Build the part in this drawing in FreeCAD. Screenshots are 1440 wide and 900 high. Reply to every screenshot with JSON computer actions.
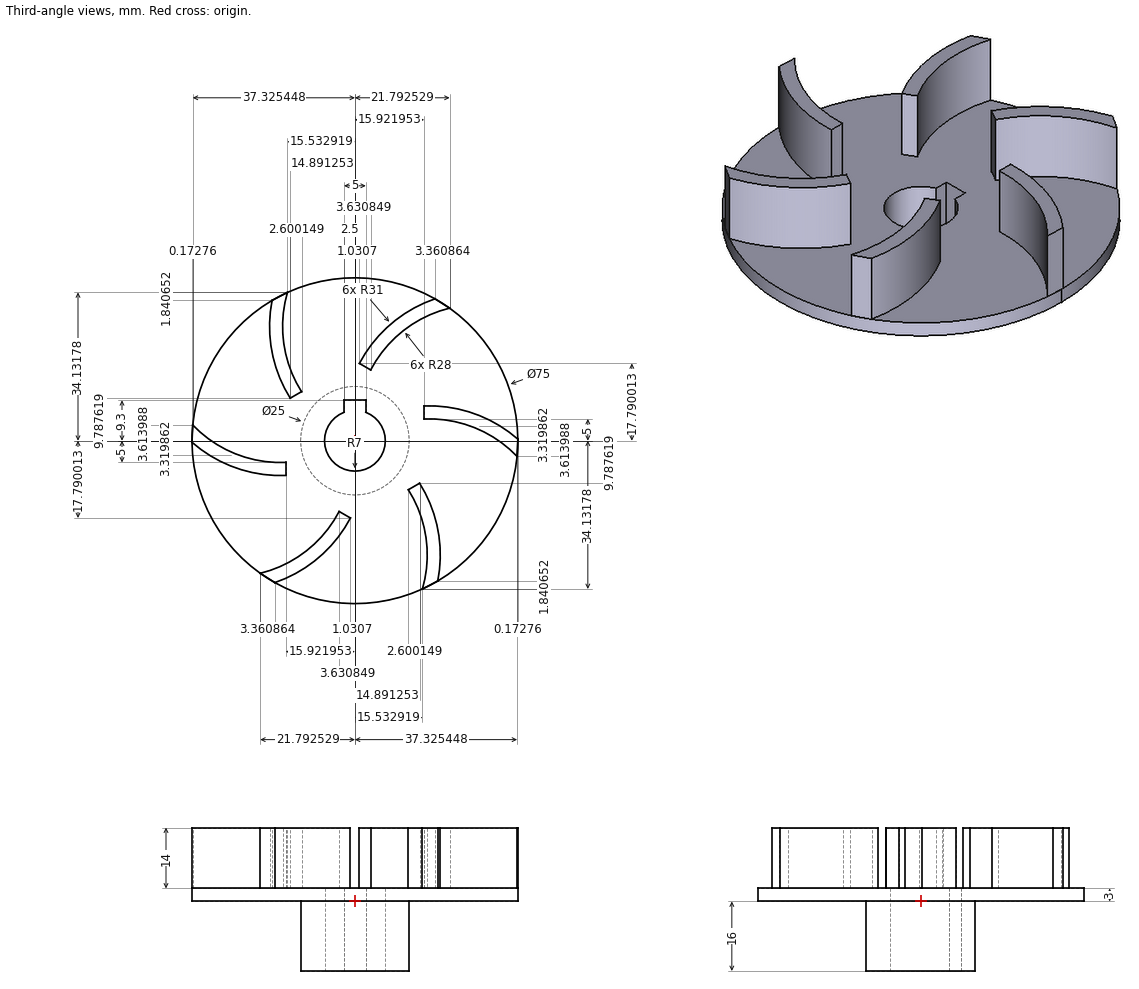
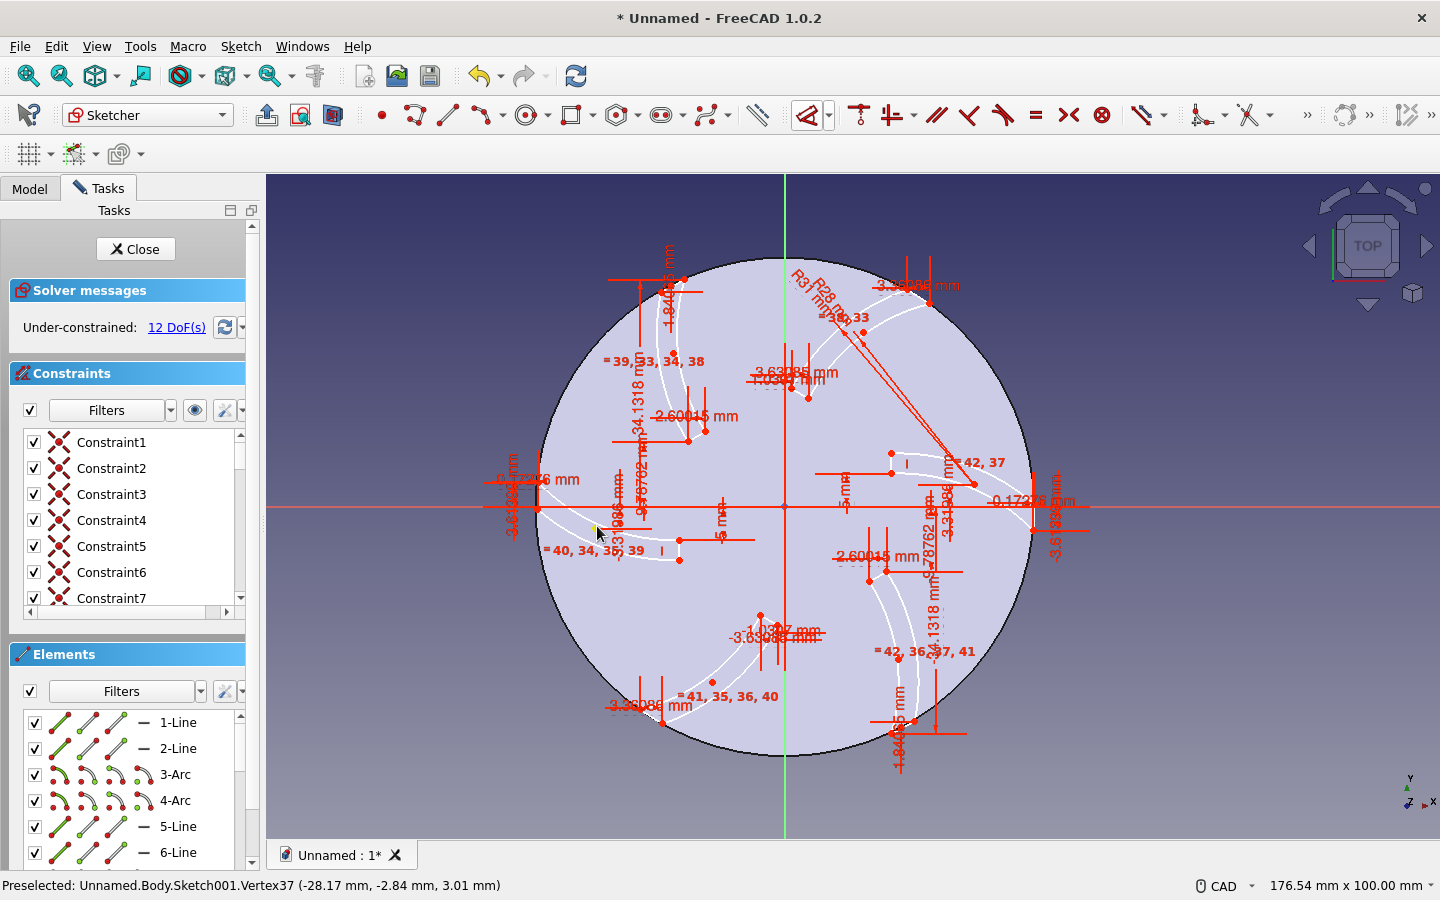
{"action": "left_click", "coordinate": [930, 304]}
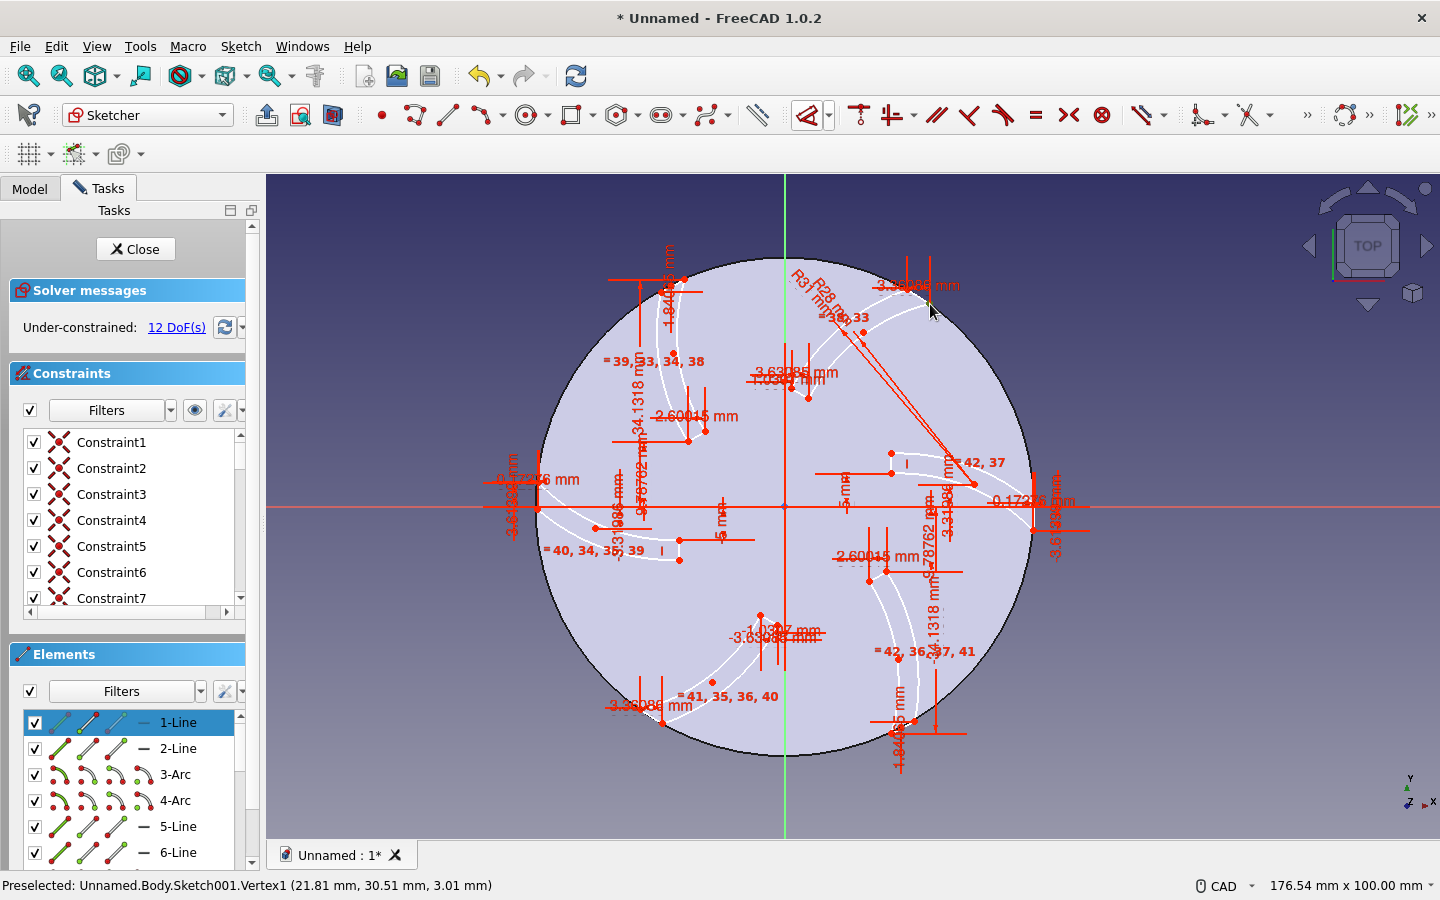
{"action": "left_click", "coordinate": [828, 116]}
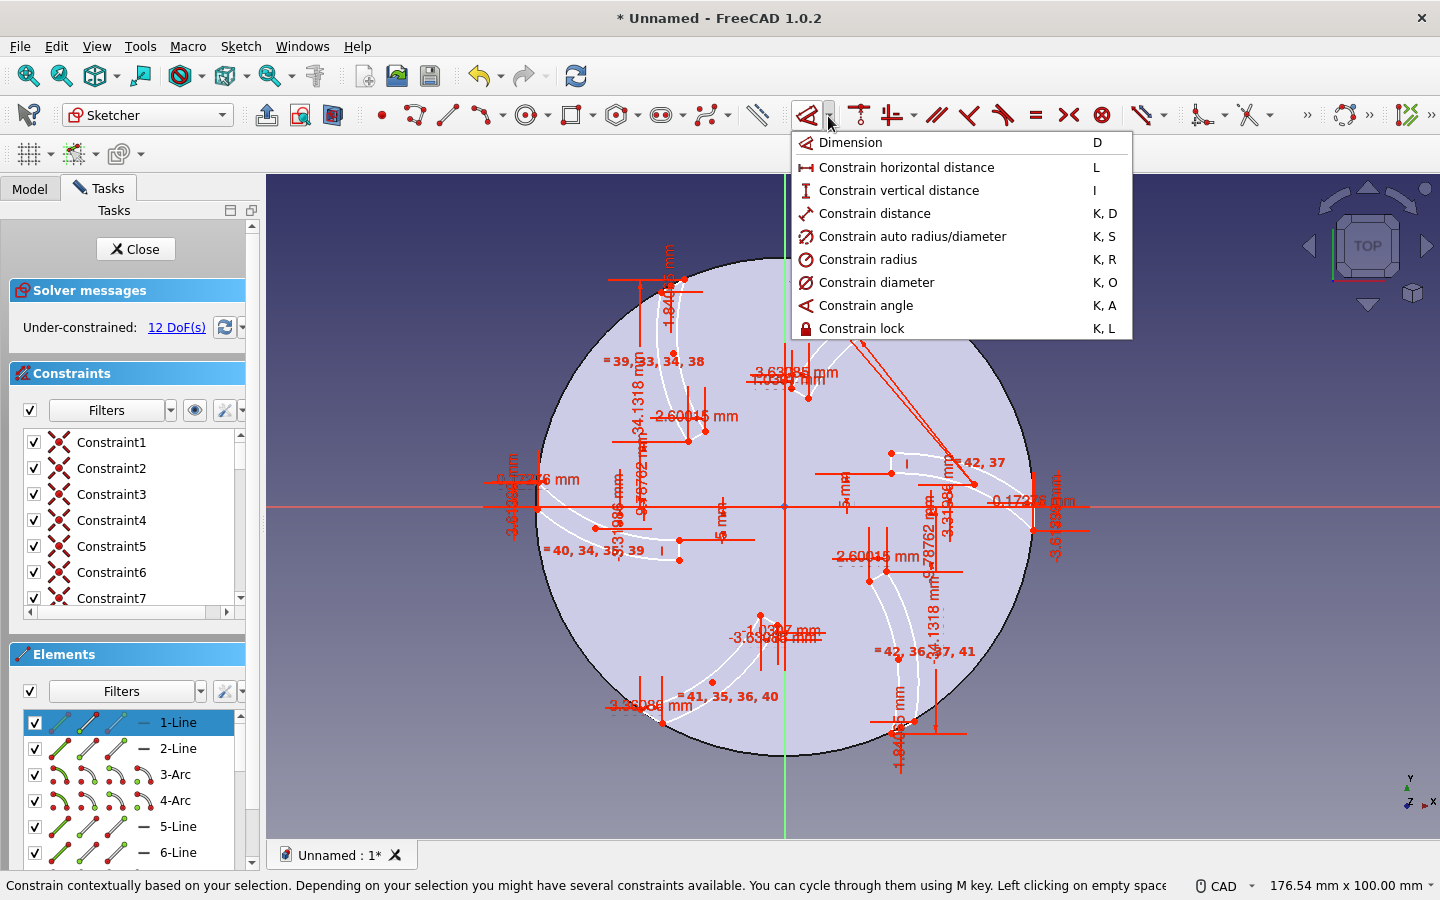
{"action": "left_click", "coordinate": [962, 168]}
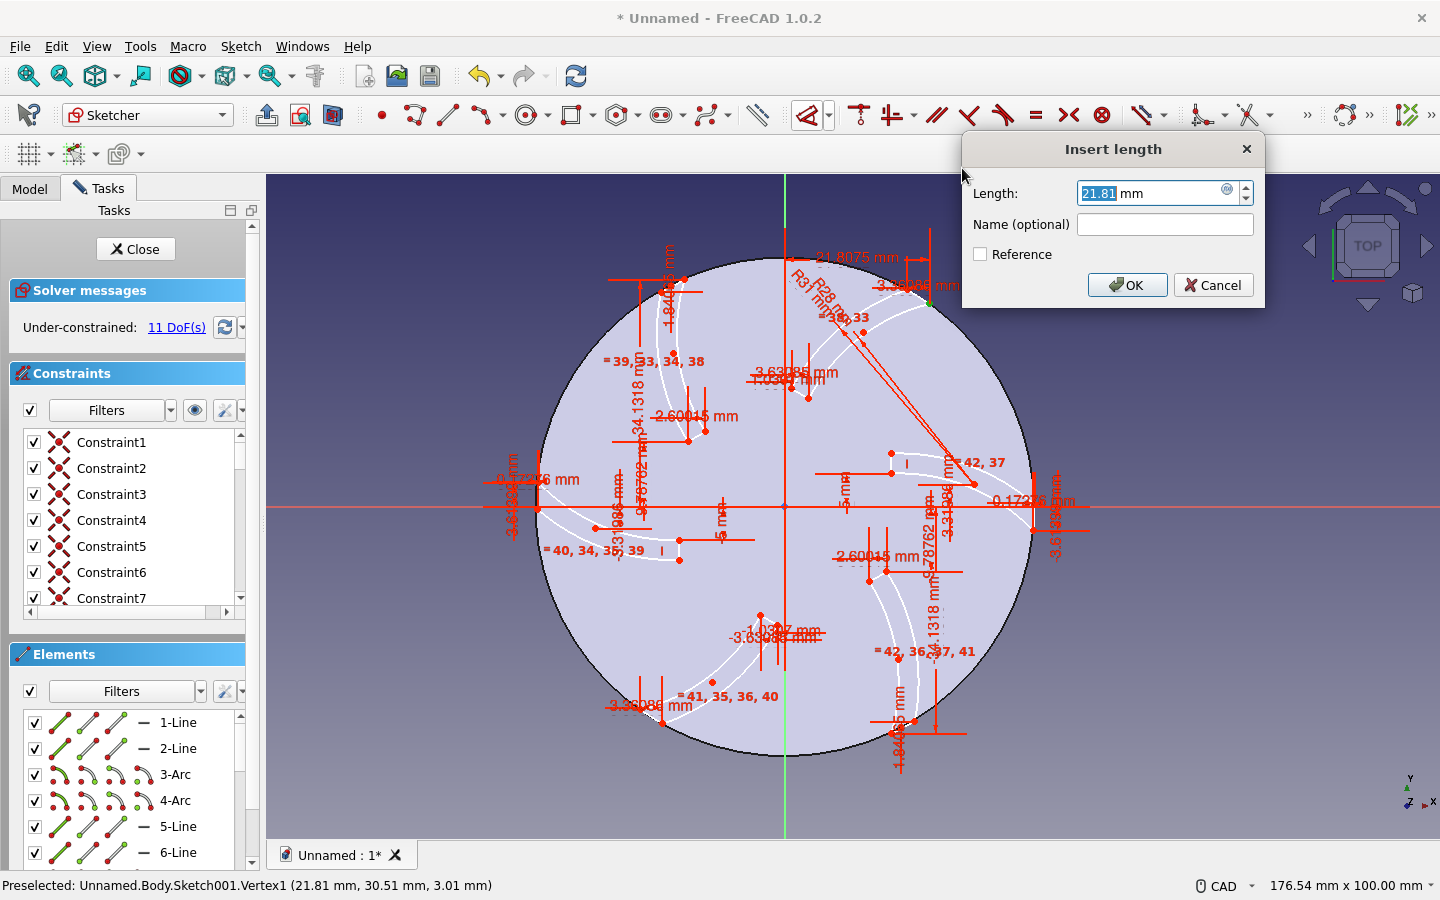
{"action": "type", "text": "21.792529"}
{"action": "key", "text": "Return"}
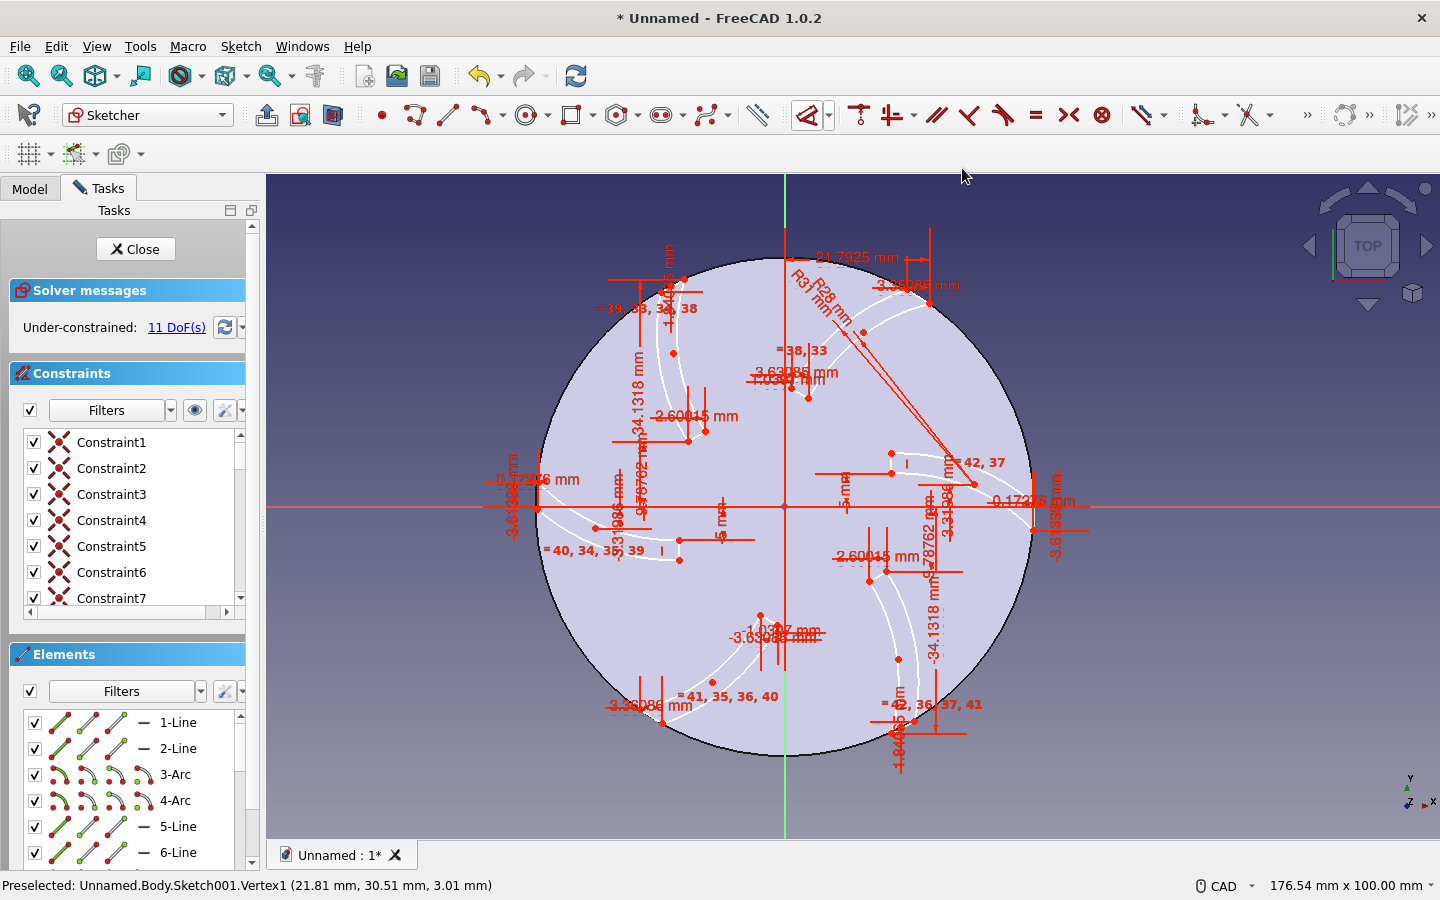
{"action": "left_click", "coordinate": [792, 389]}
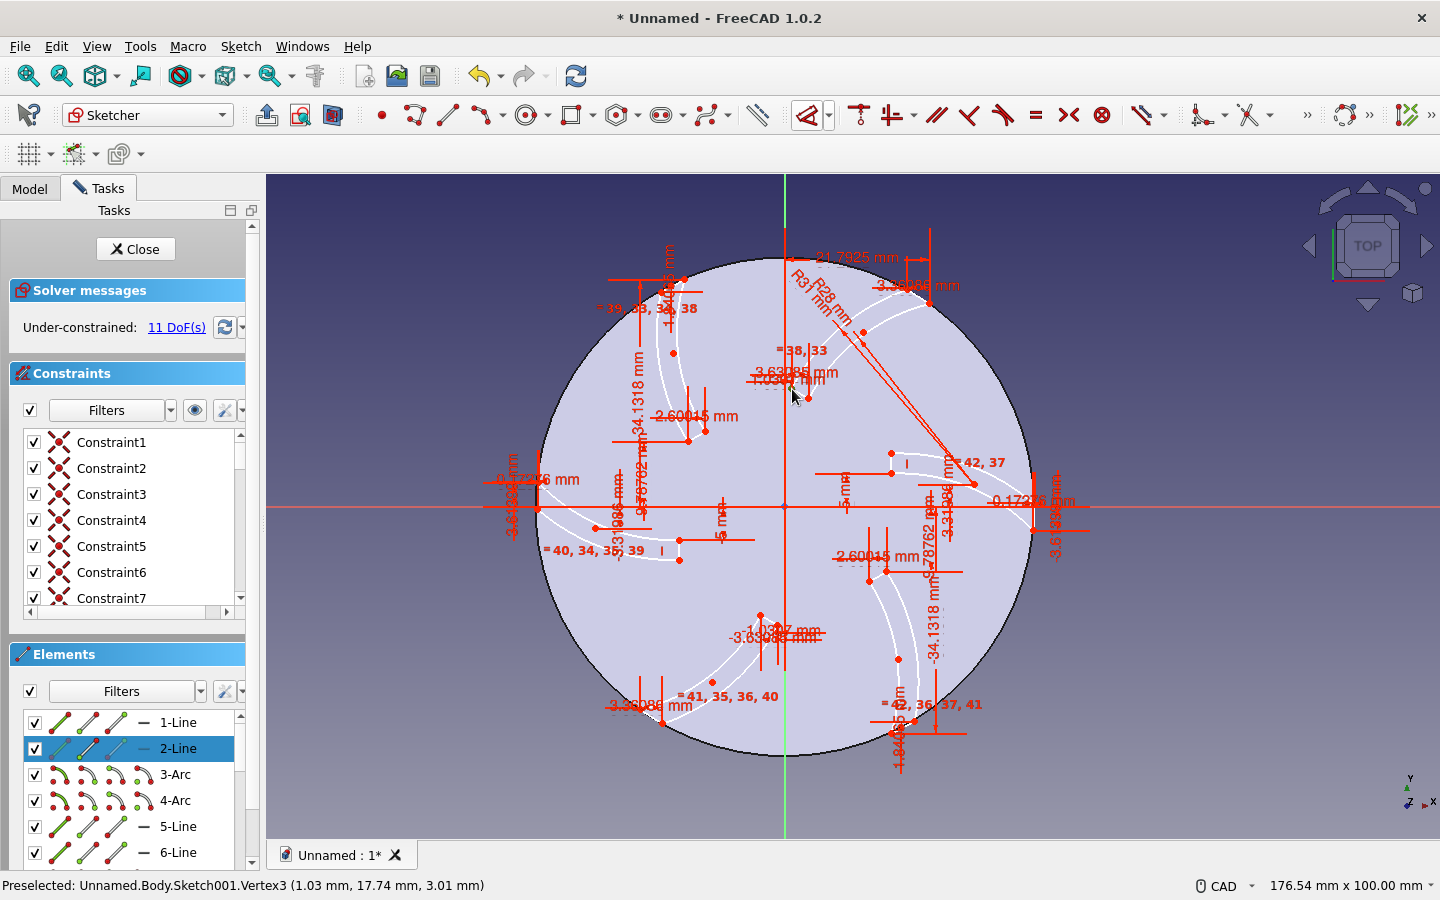
{"action": "key", "text": "i"}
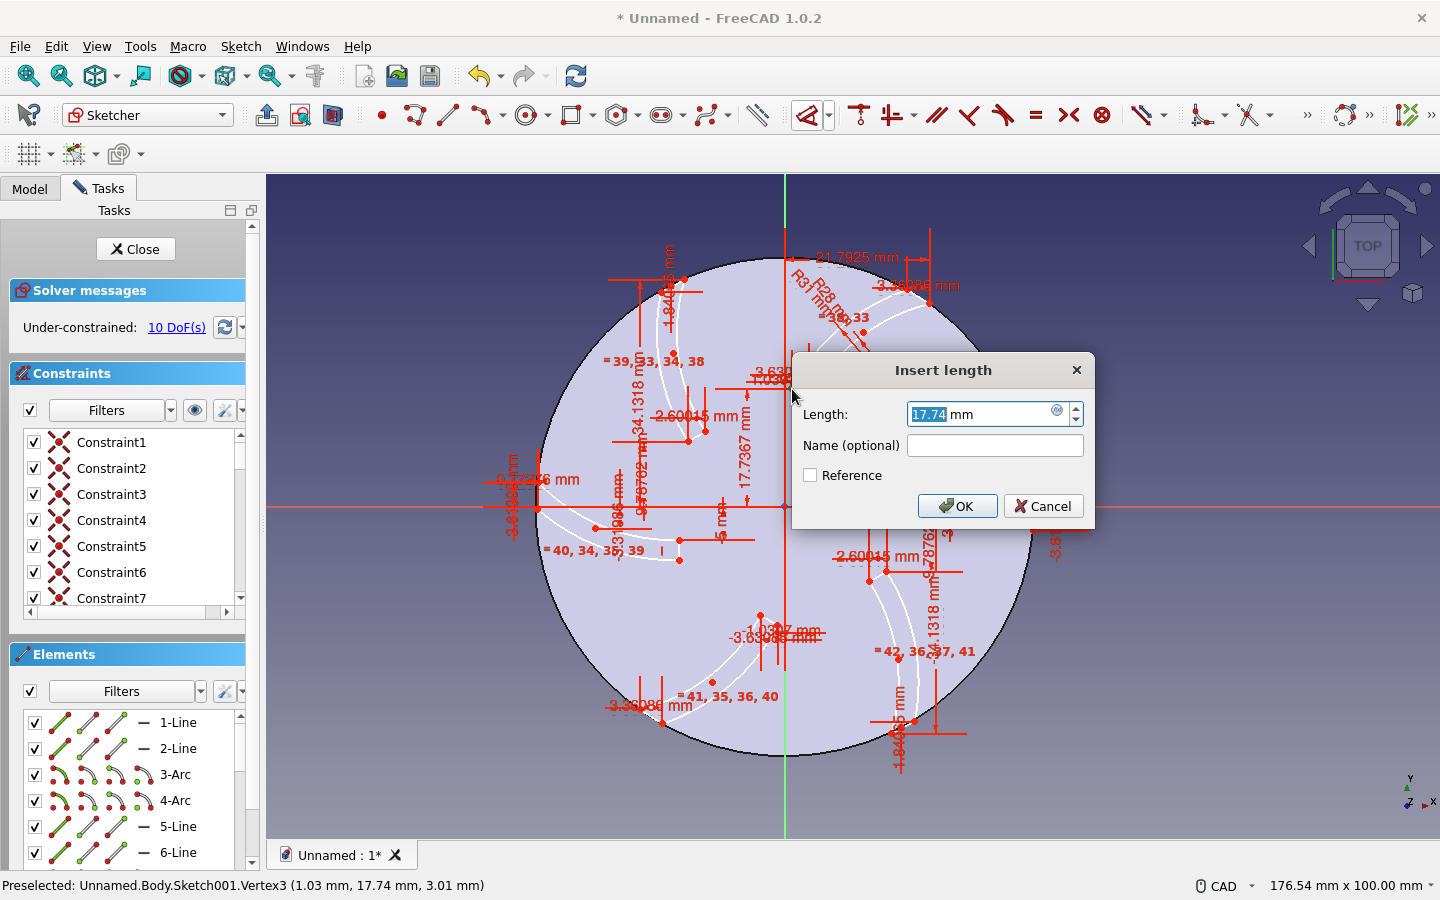
{"action": "type", "text": "17.790013"}
{"action": "key", "text": "Return"}